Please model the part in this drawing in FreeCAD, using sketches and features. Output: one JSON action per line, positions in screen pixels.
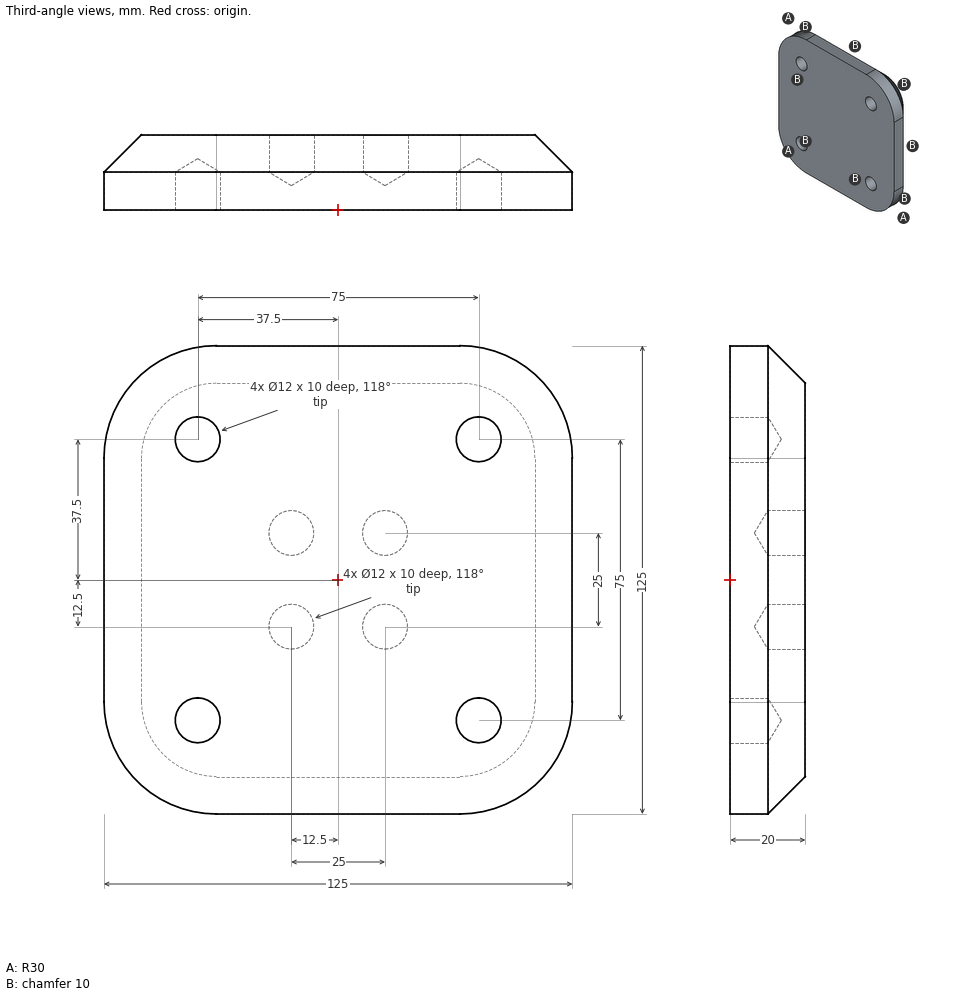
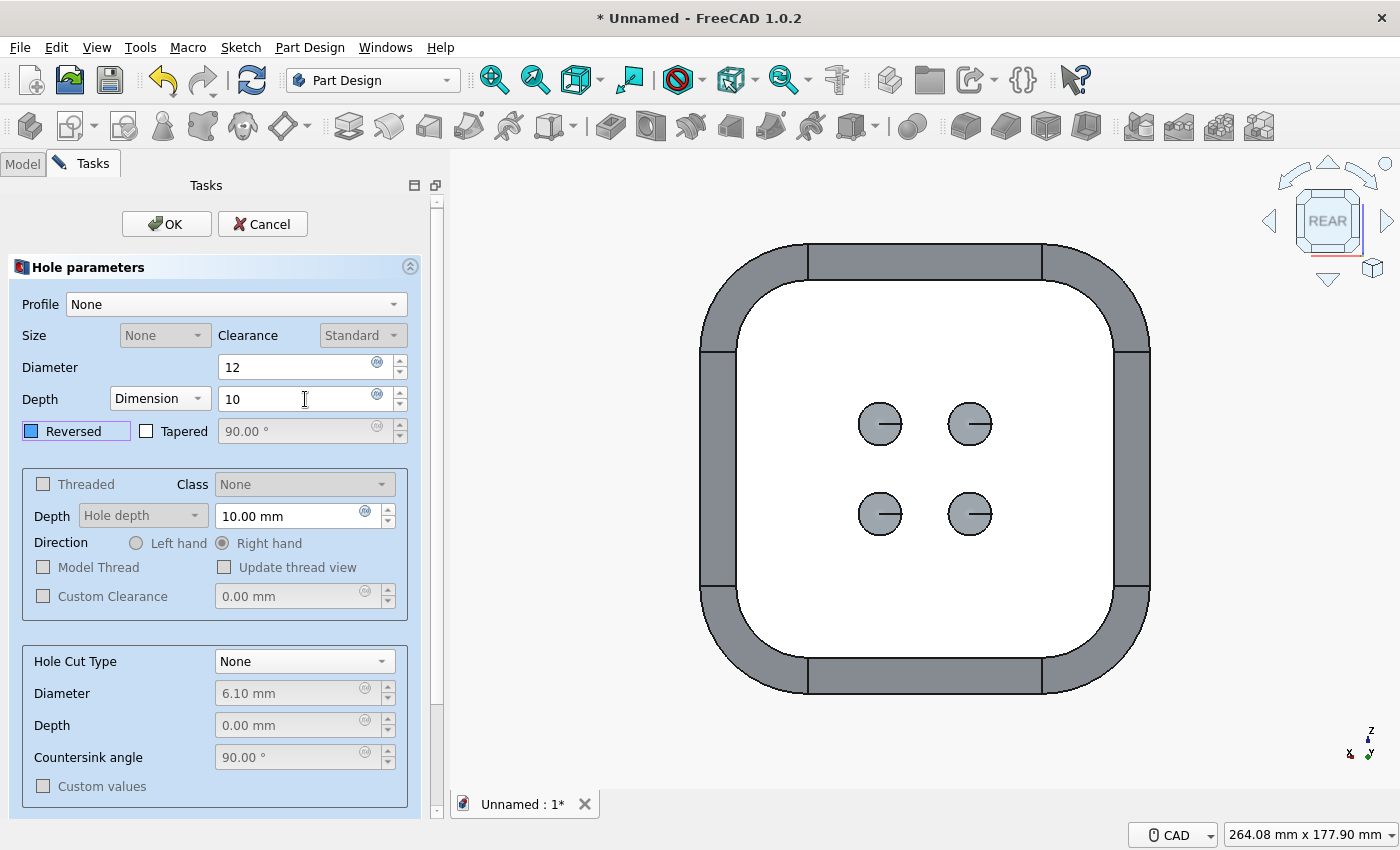
{"action": "left_click", "coordinate": [167, 224]}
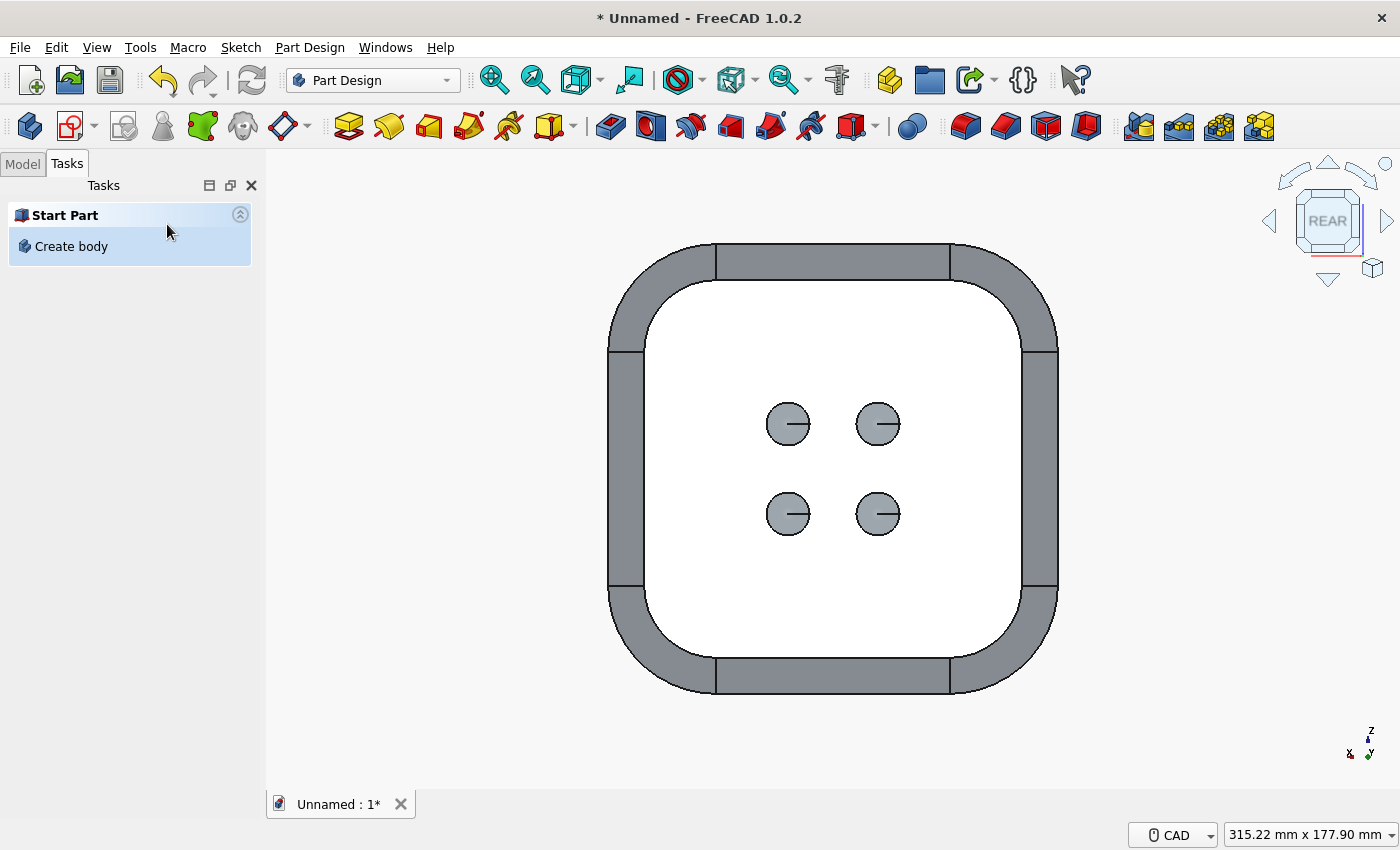
{"action": "key", "text": "0"}